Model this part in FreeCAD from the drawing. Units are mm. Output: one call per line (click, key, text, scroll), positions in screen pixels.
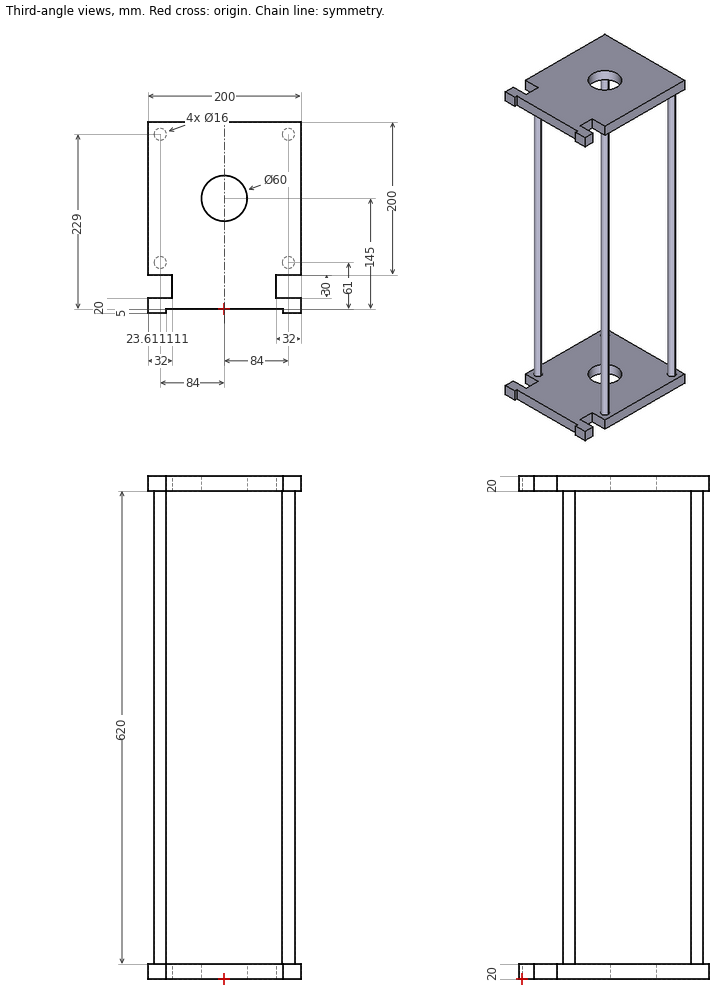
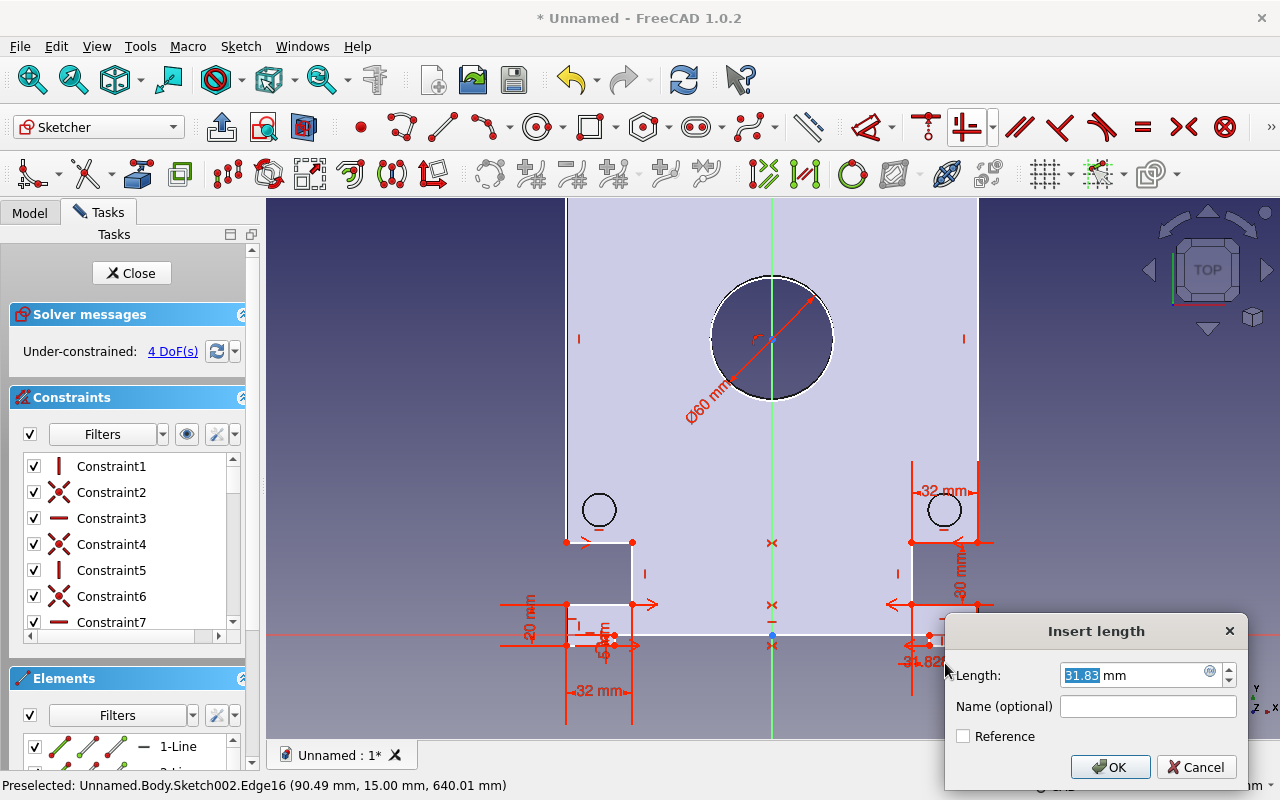
text(32)
key(Return)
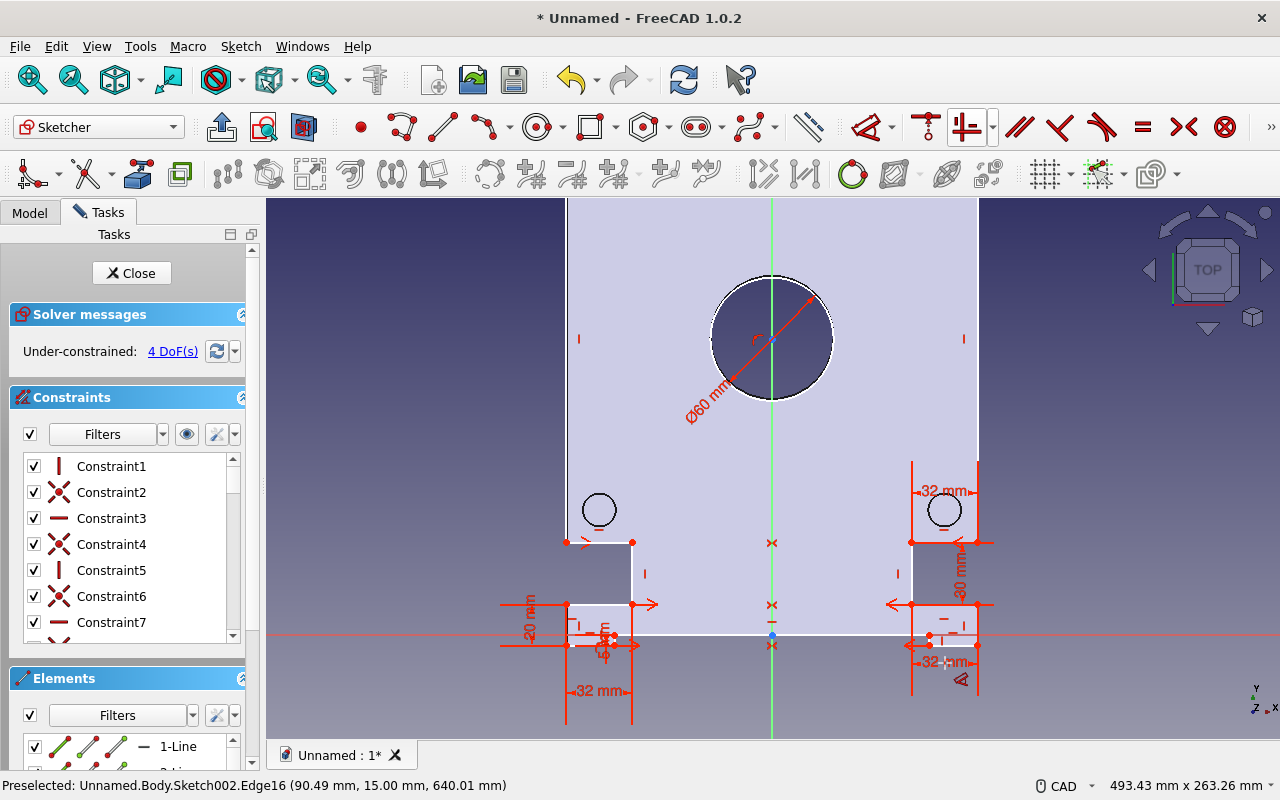
click(978, 420)
click(1012, 384)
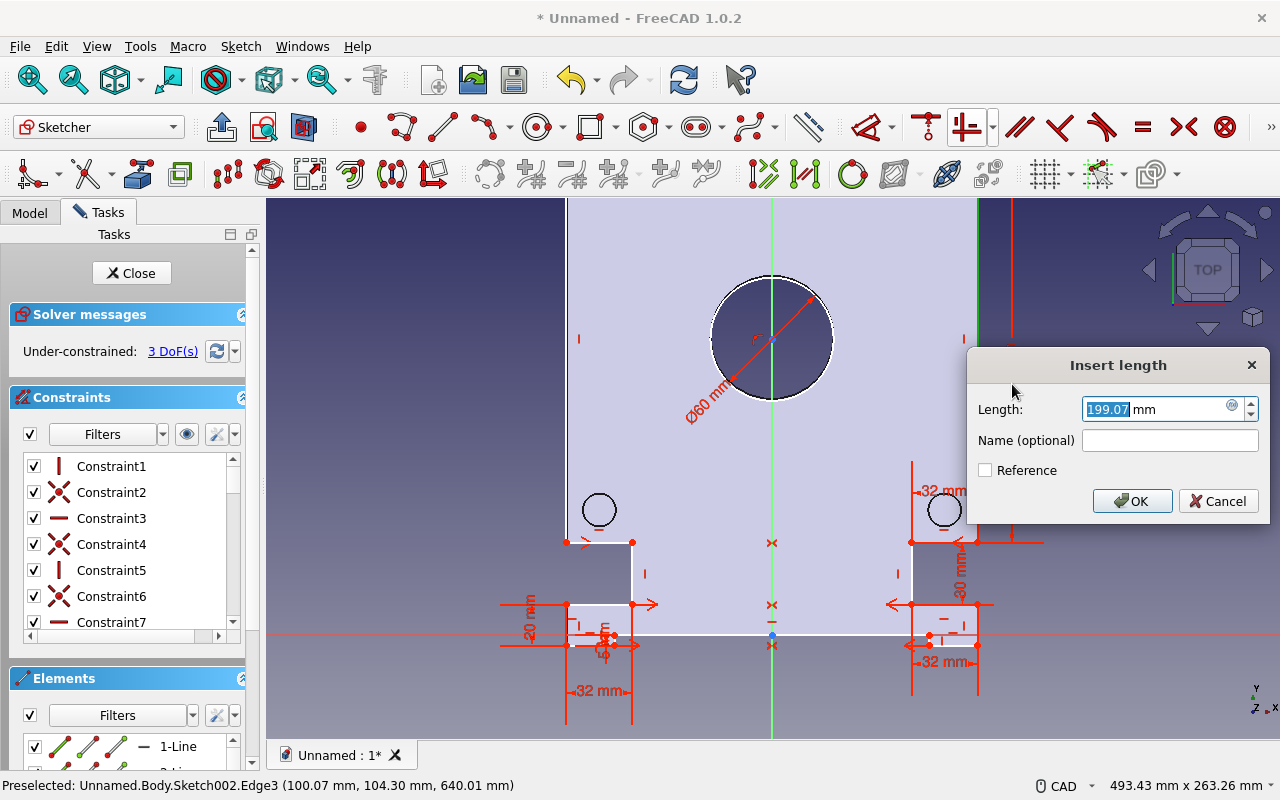
text(200)
key(Return)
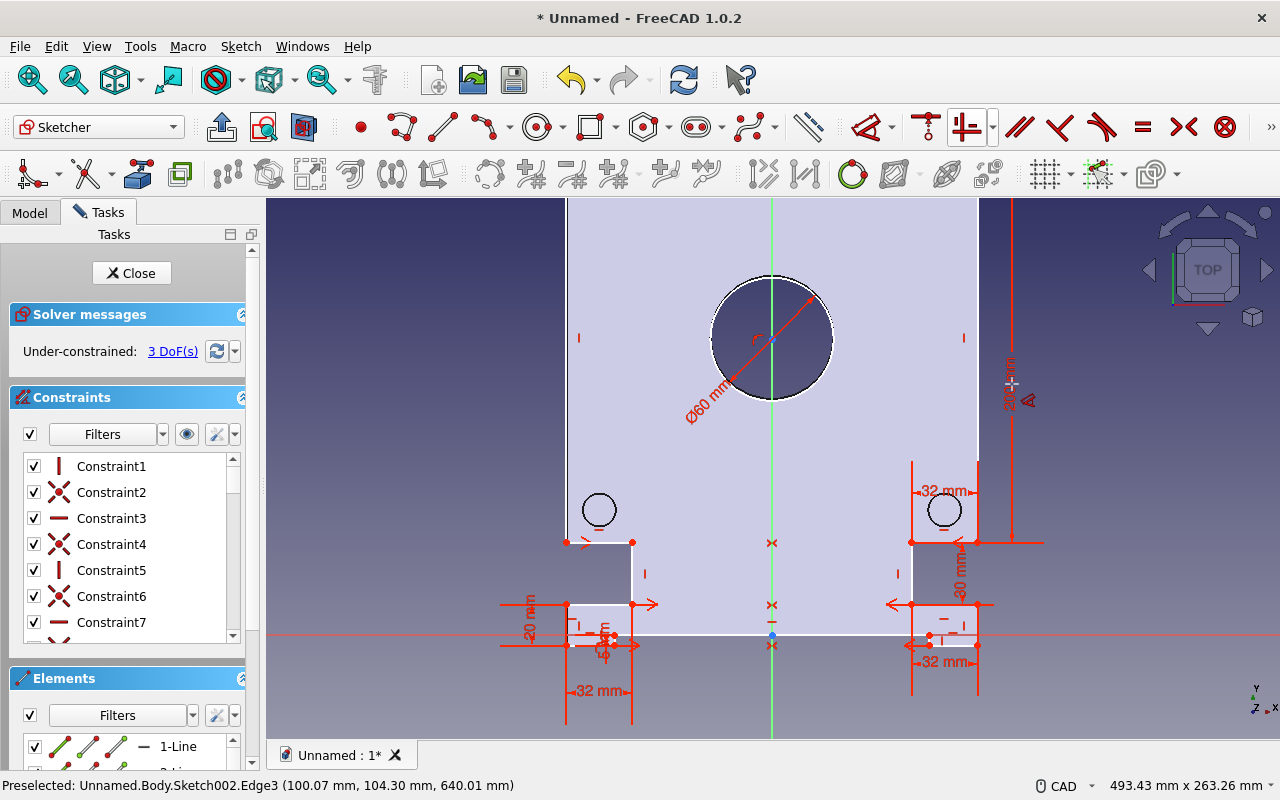
scroll(567, 631, down, 2)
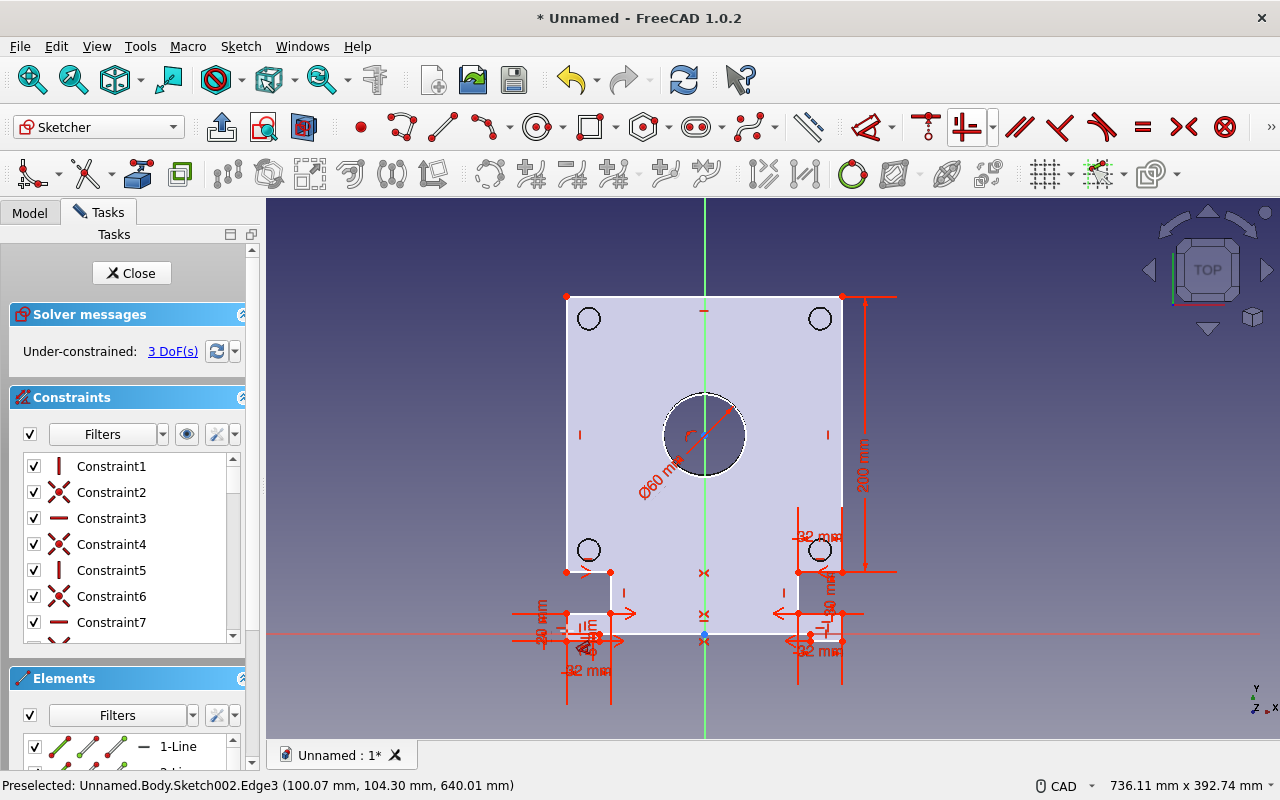
click(760, 297)
click(641, 263)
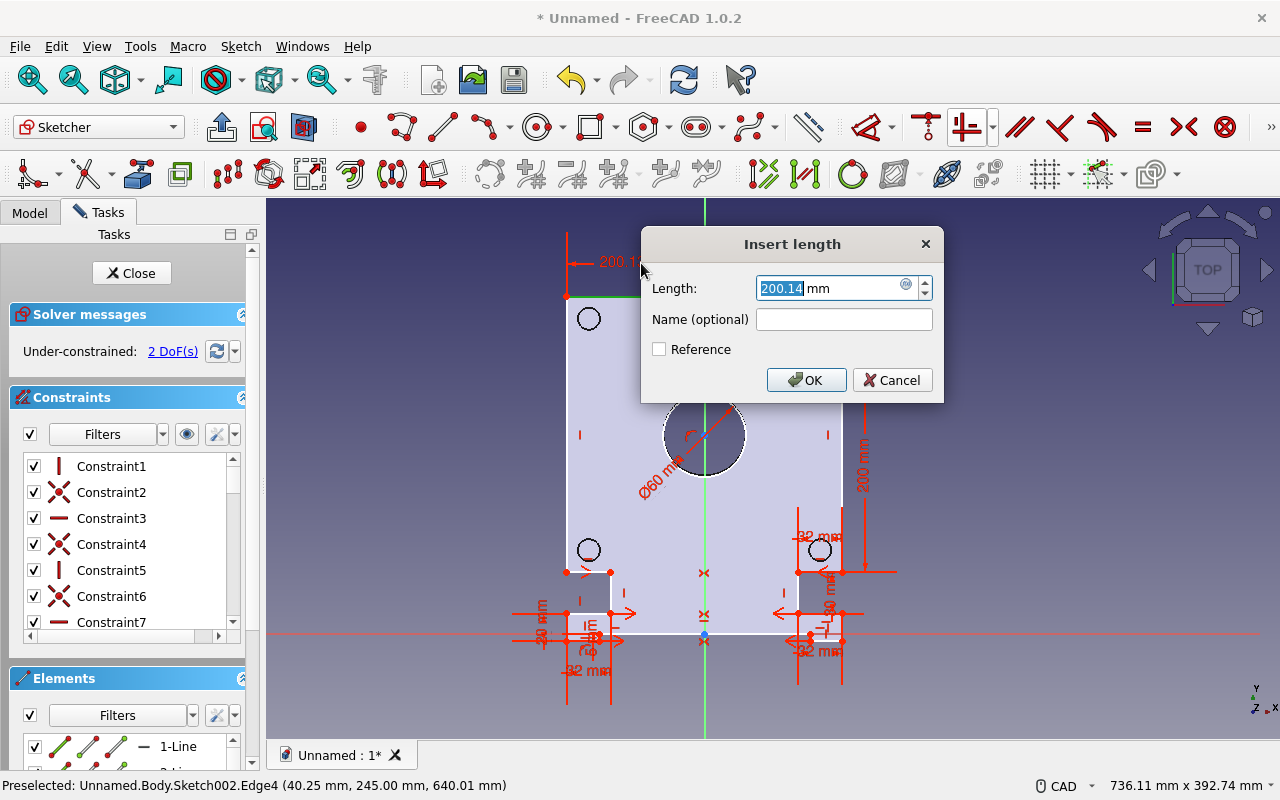
text(200)
key(Return)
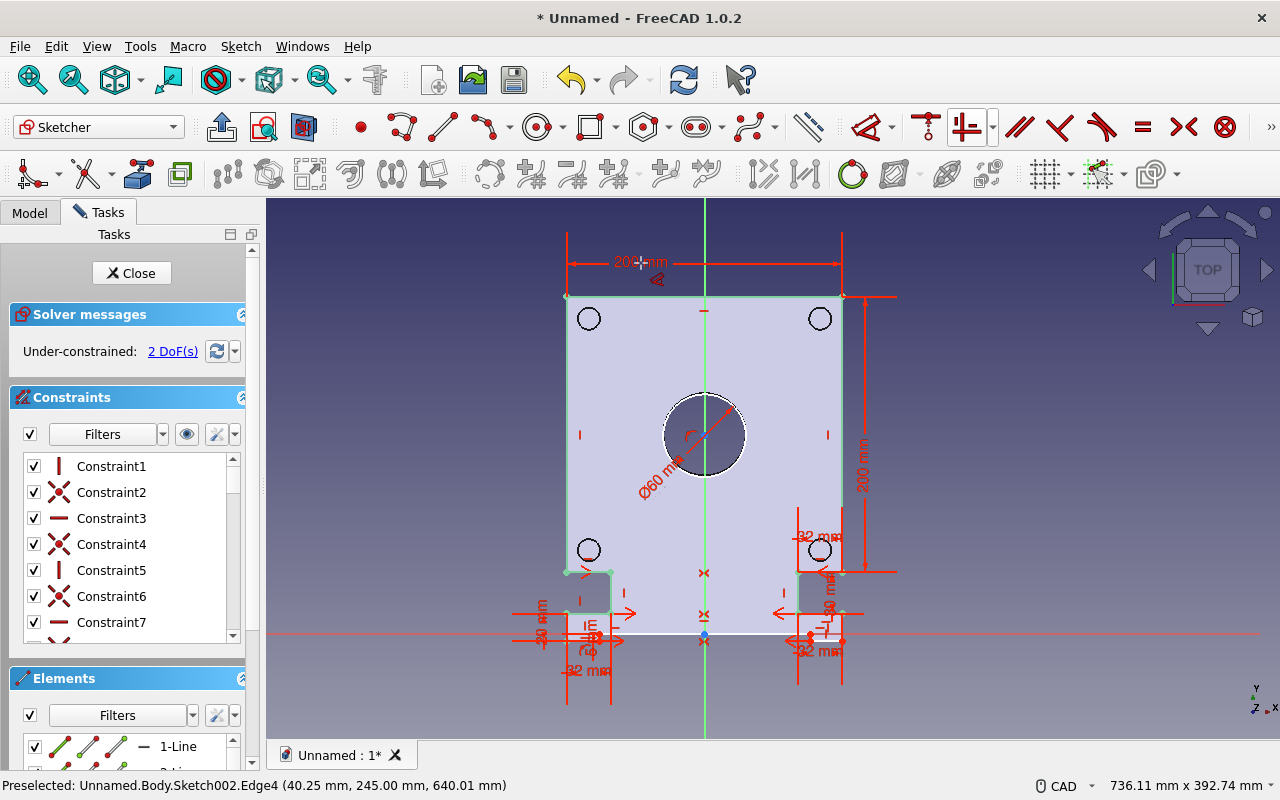
click(705, 436)
click(739, 535)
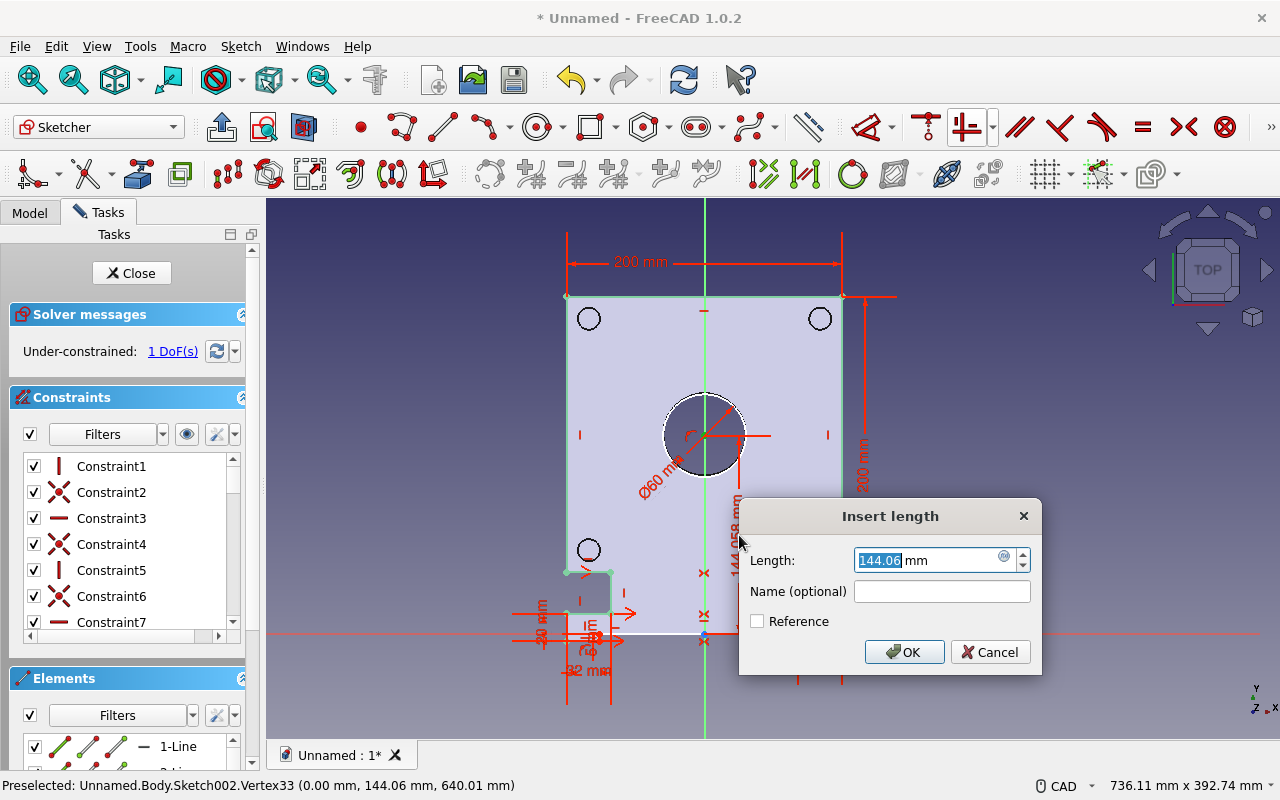
text(145)
key(Return)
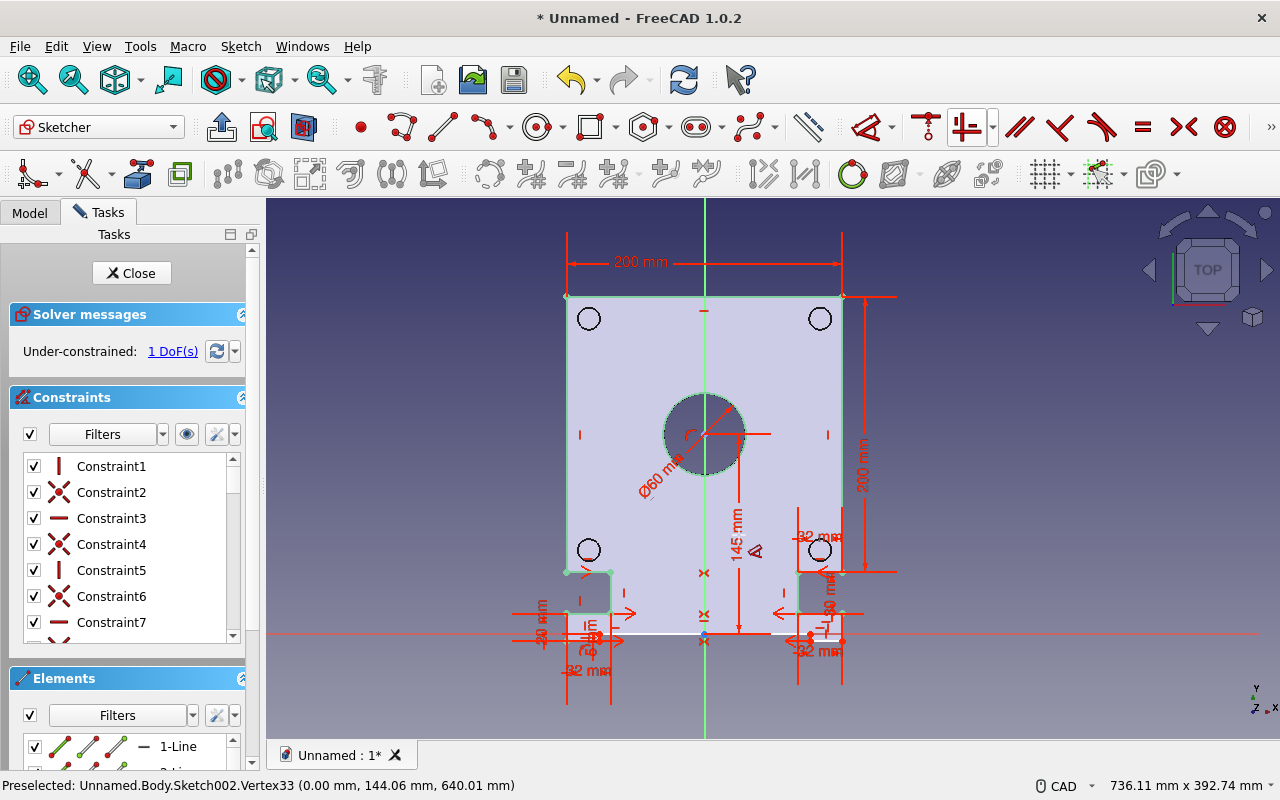
scroll(576, 641, up, 4)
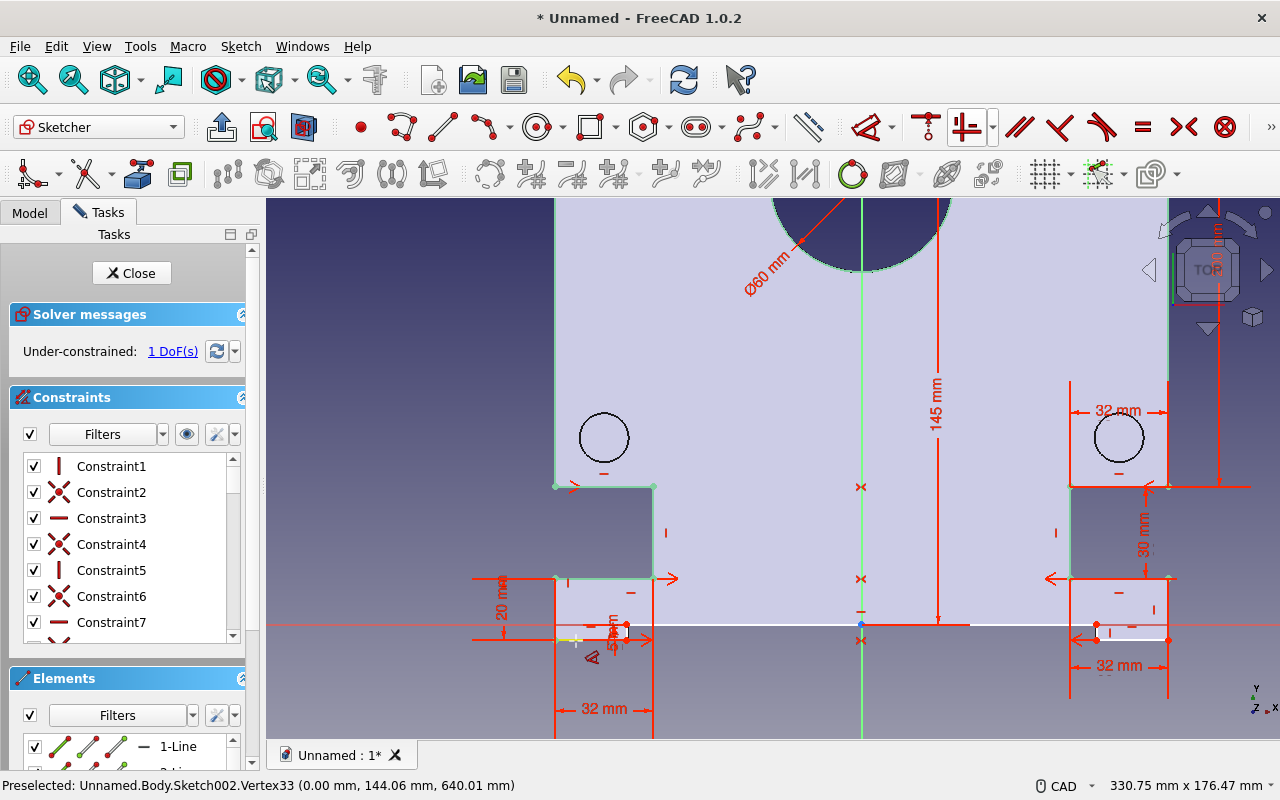
click(577, 640)
click(591, 674)